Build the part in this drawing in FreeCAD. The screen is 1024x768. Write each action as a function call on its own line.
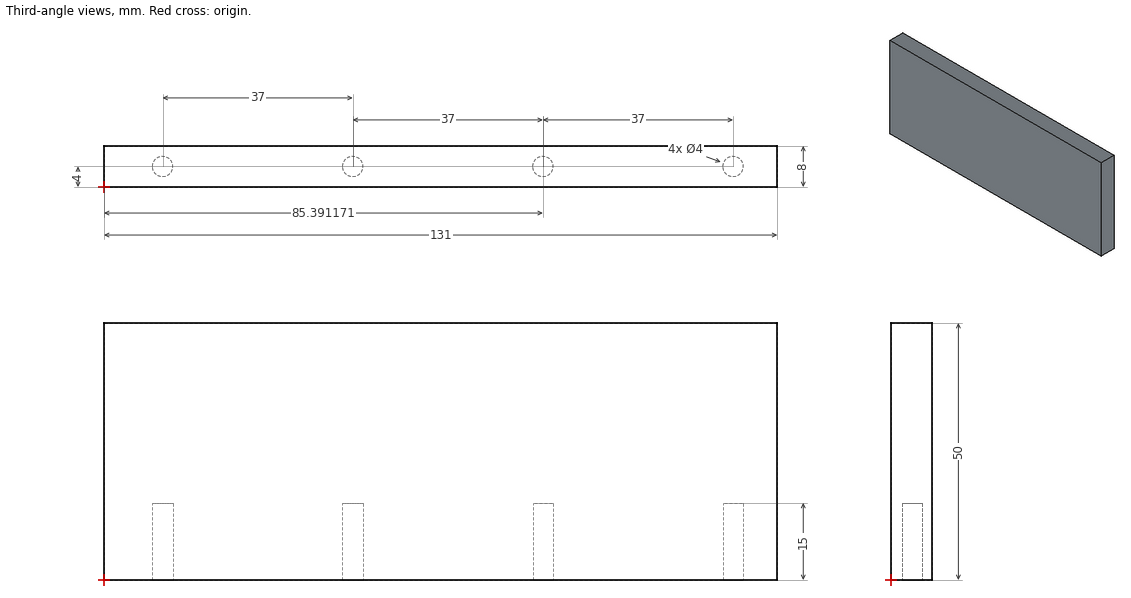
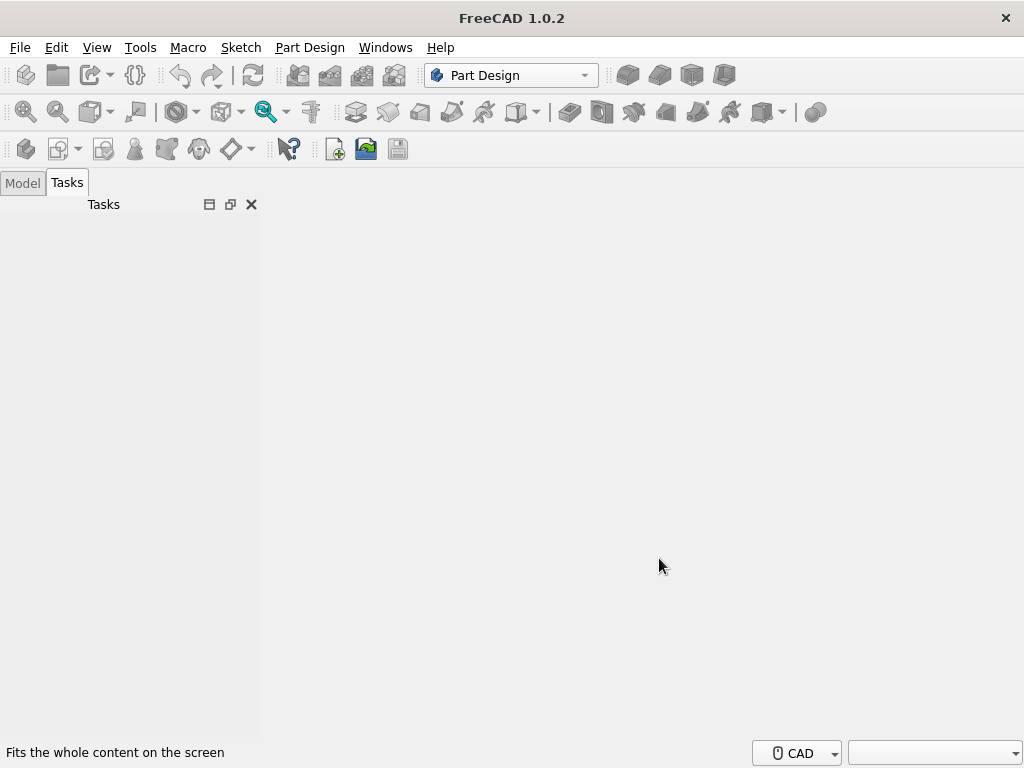
click(334, 150)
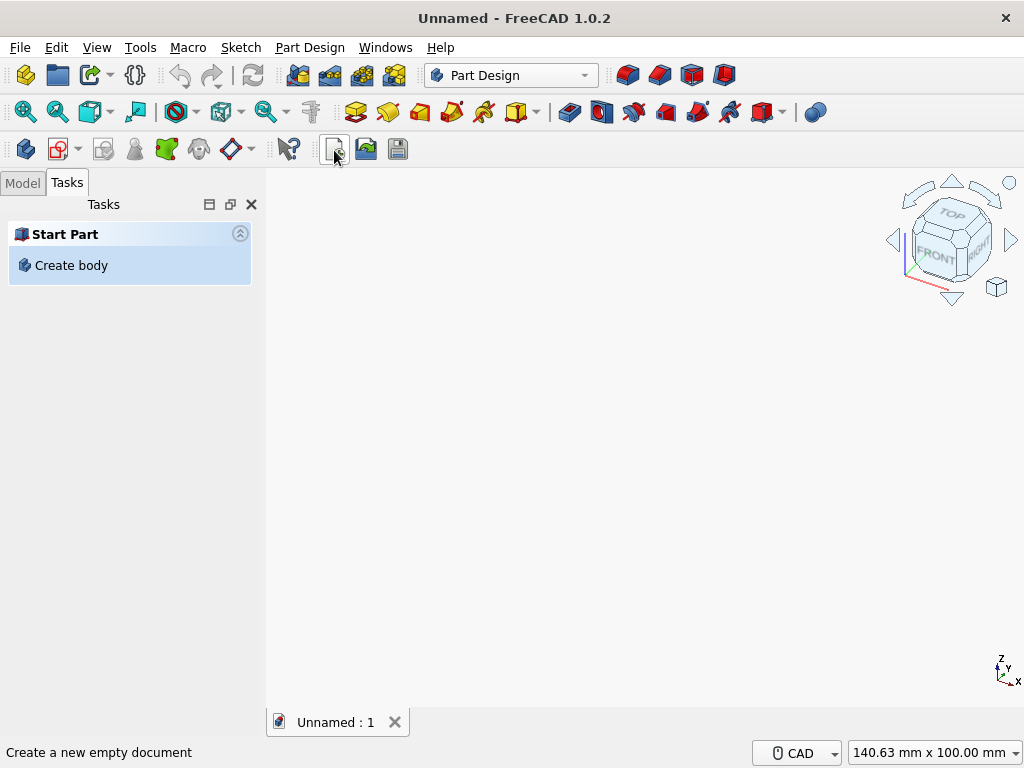
click(58, 150)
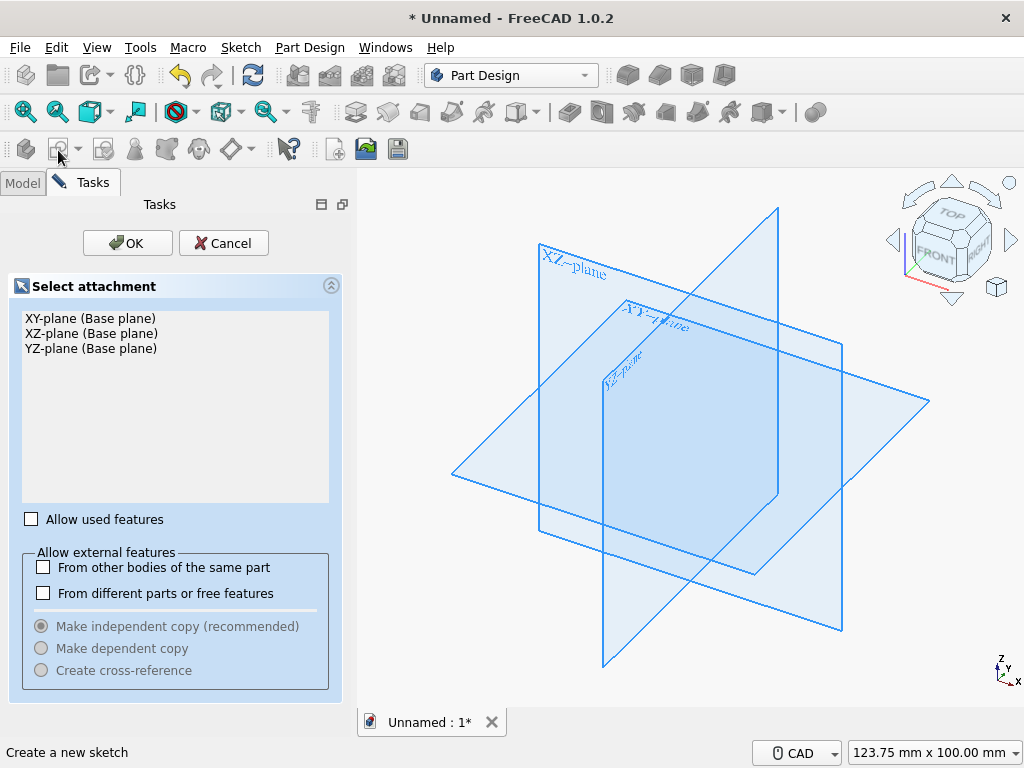
click(82, 318)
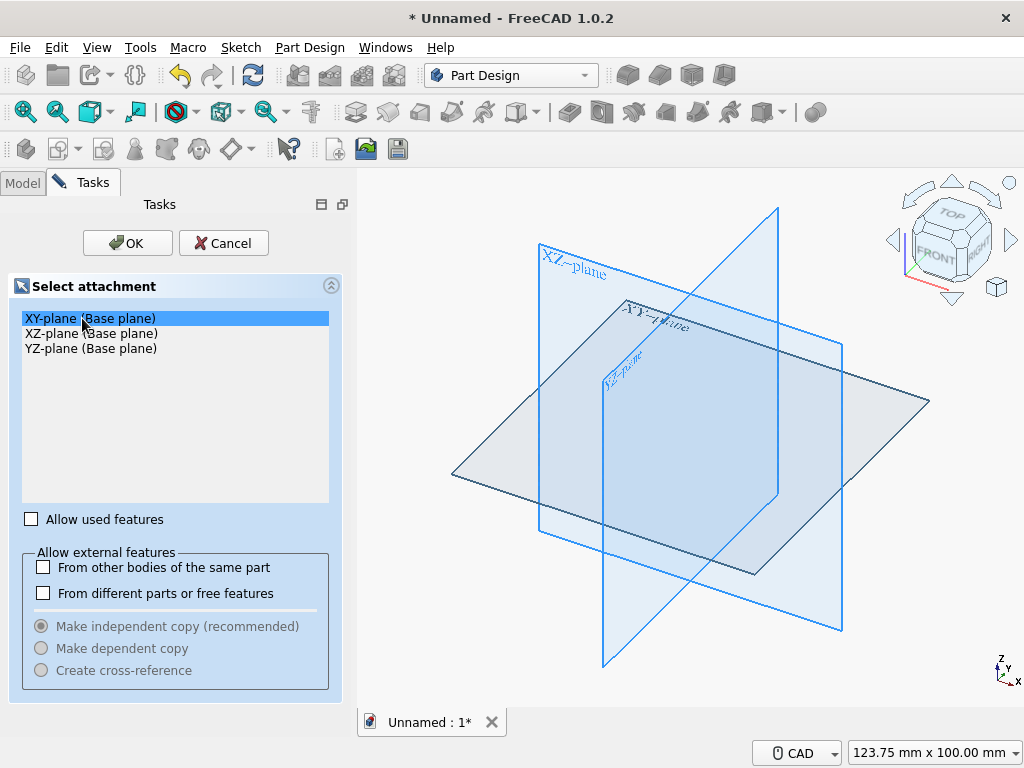
click(128, 243)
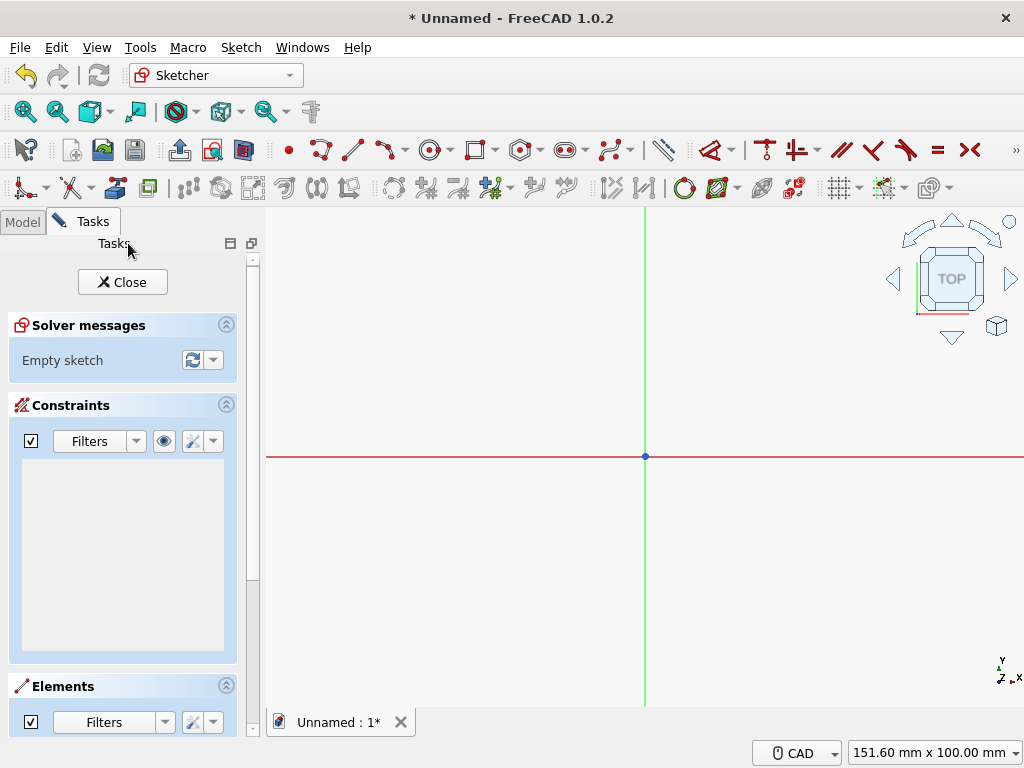
scroll(294, 473, down, 4)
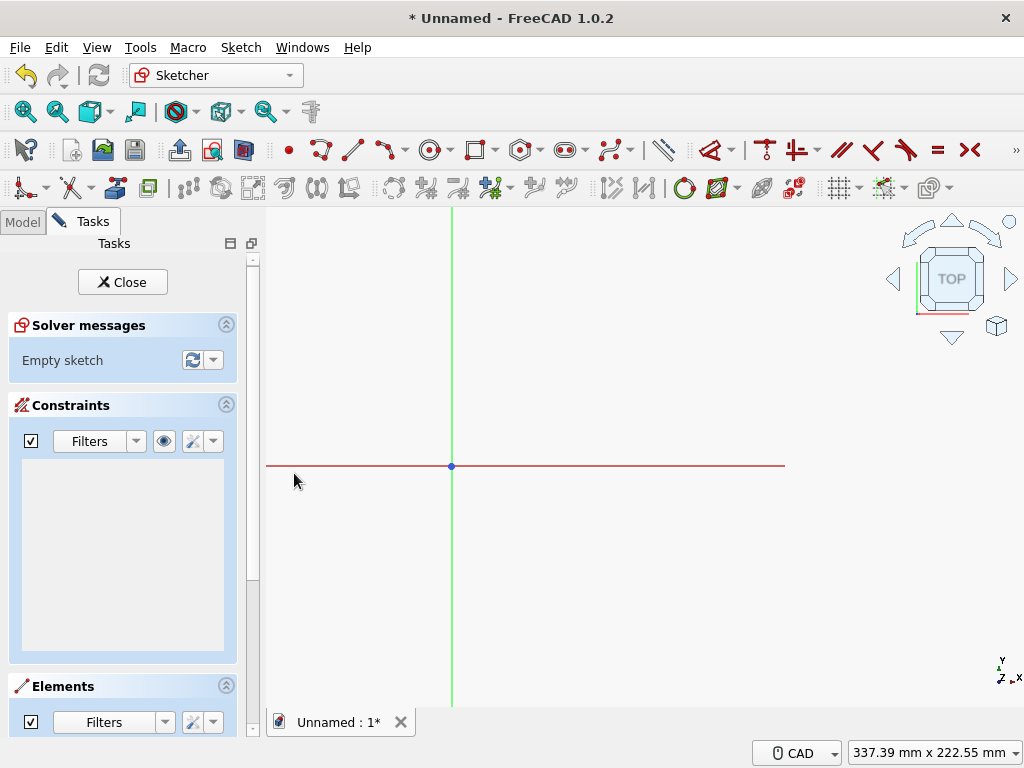
scroll(644, 457, up, 2)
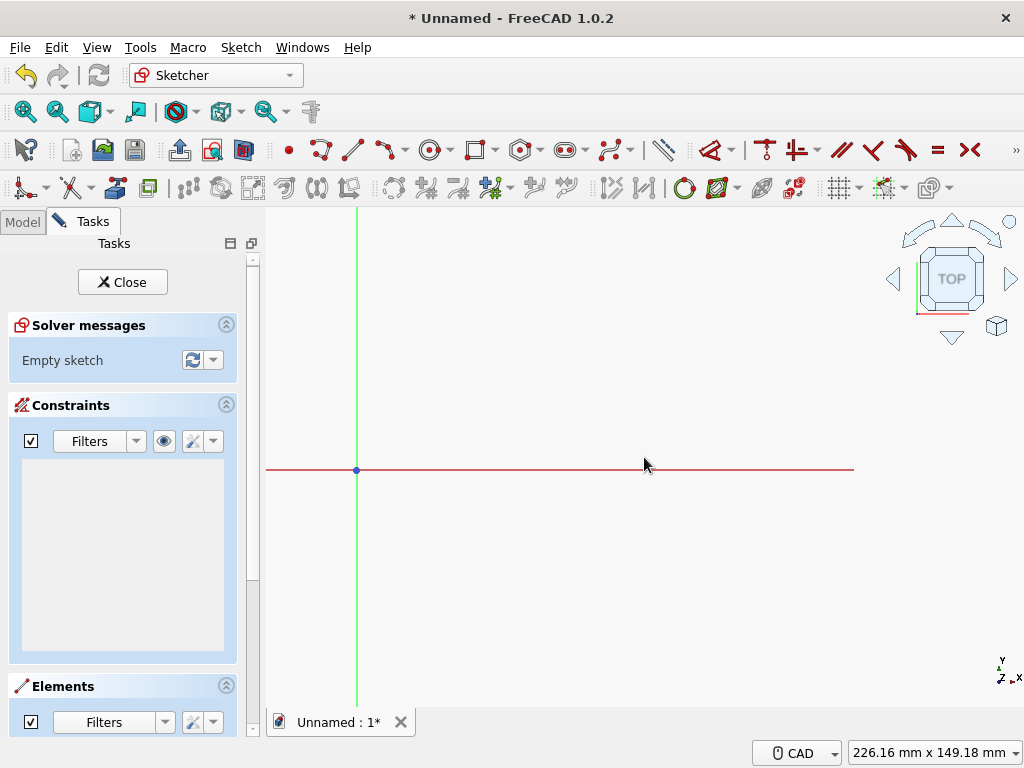
click(476, 150)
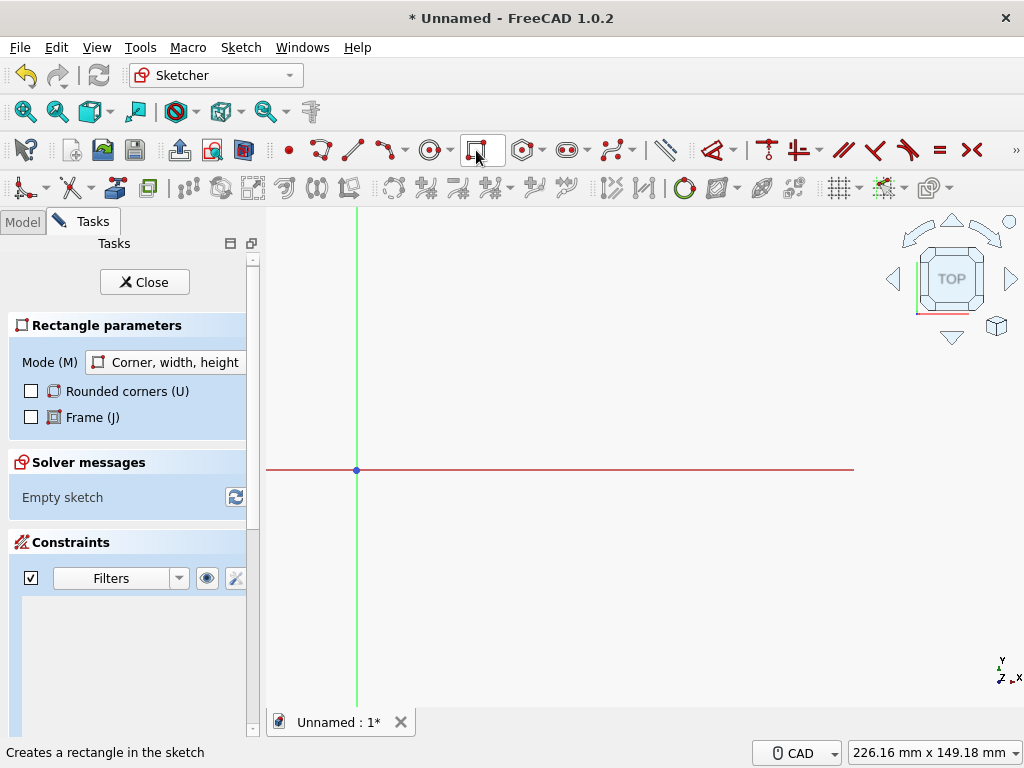
click(357, 470)
click(796, 444)
key(Escape)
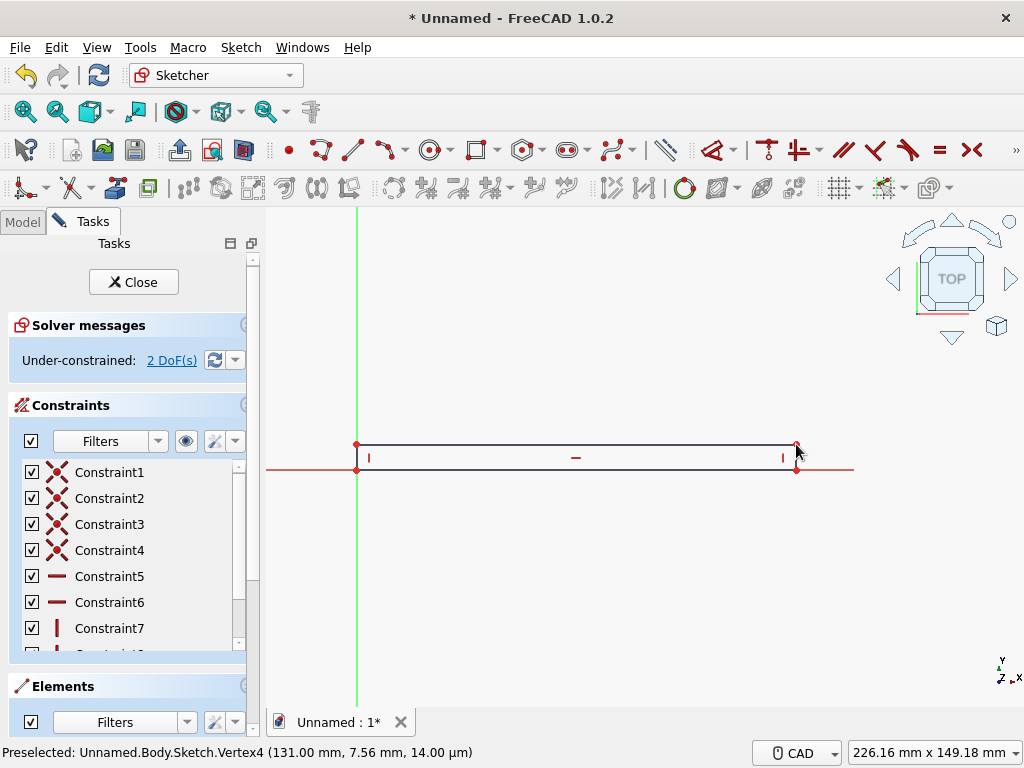
click(712, 150)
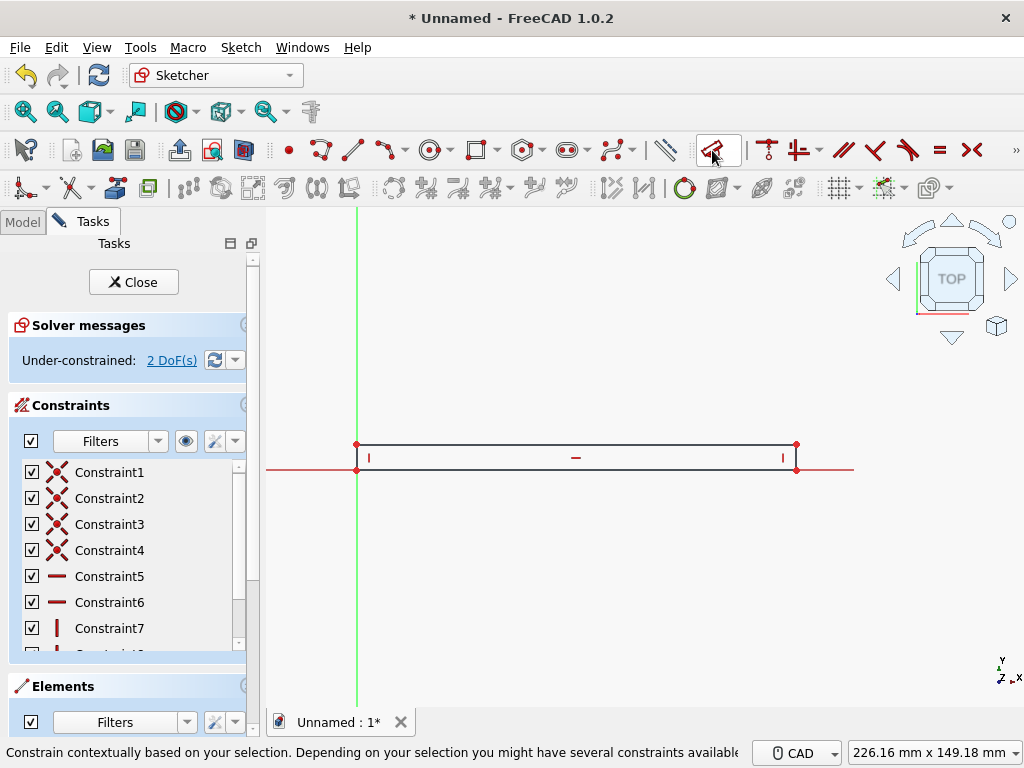
scroll(796, 460, up, 2)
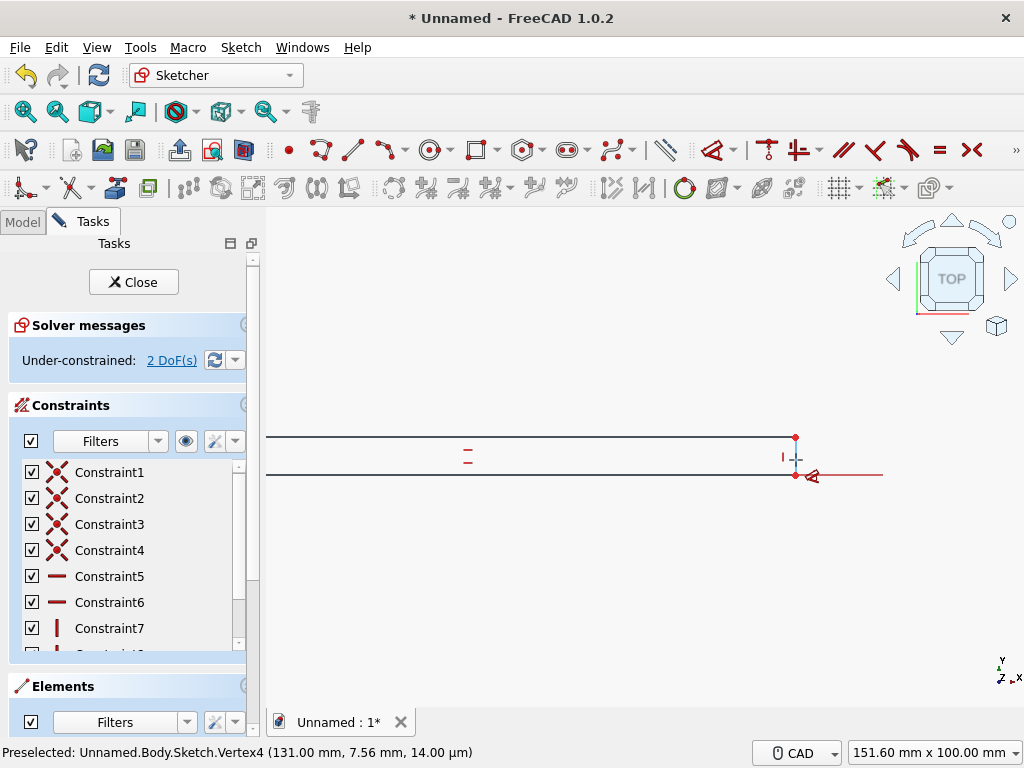
click(796, 460)
click(830, 456)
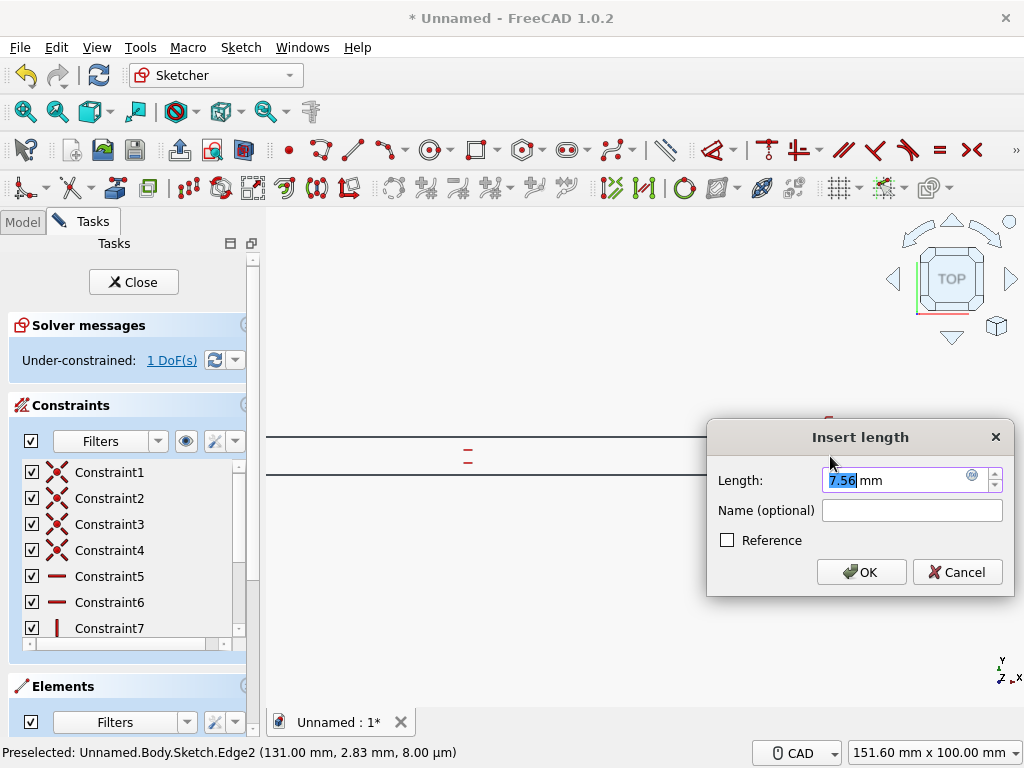
text(8)
key(Return)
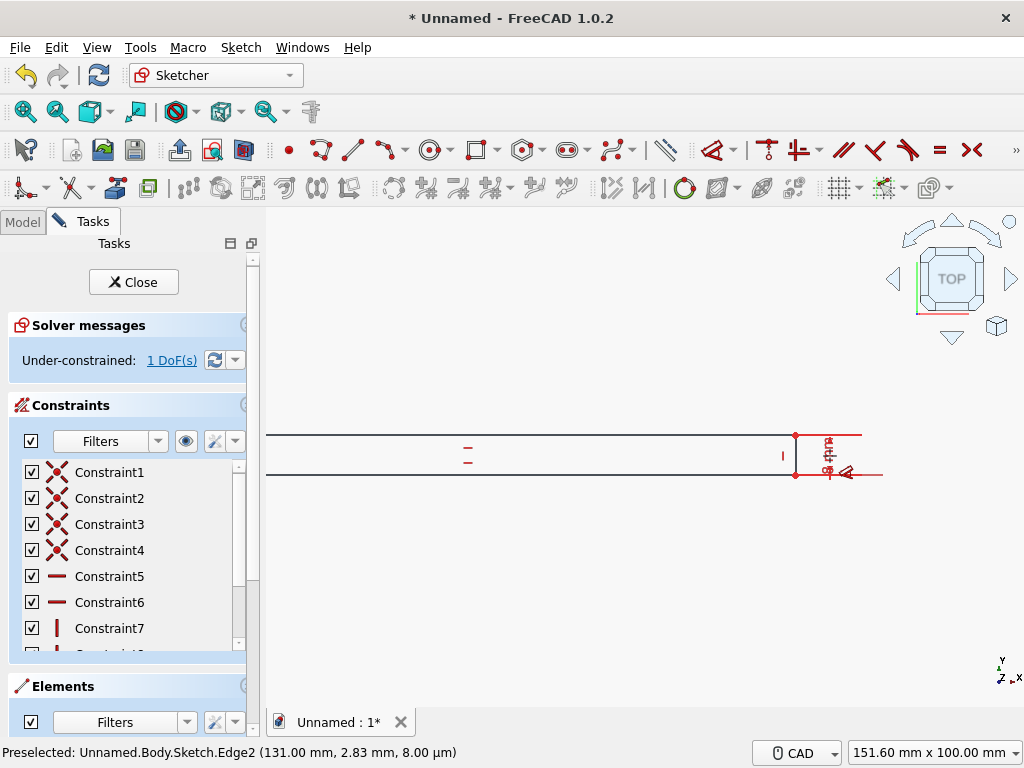
click(337, 475)
click(545, 509)